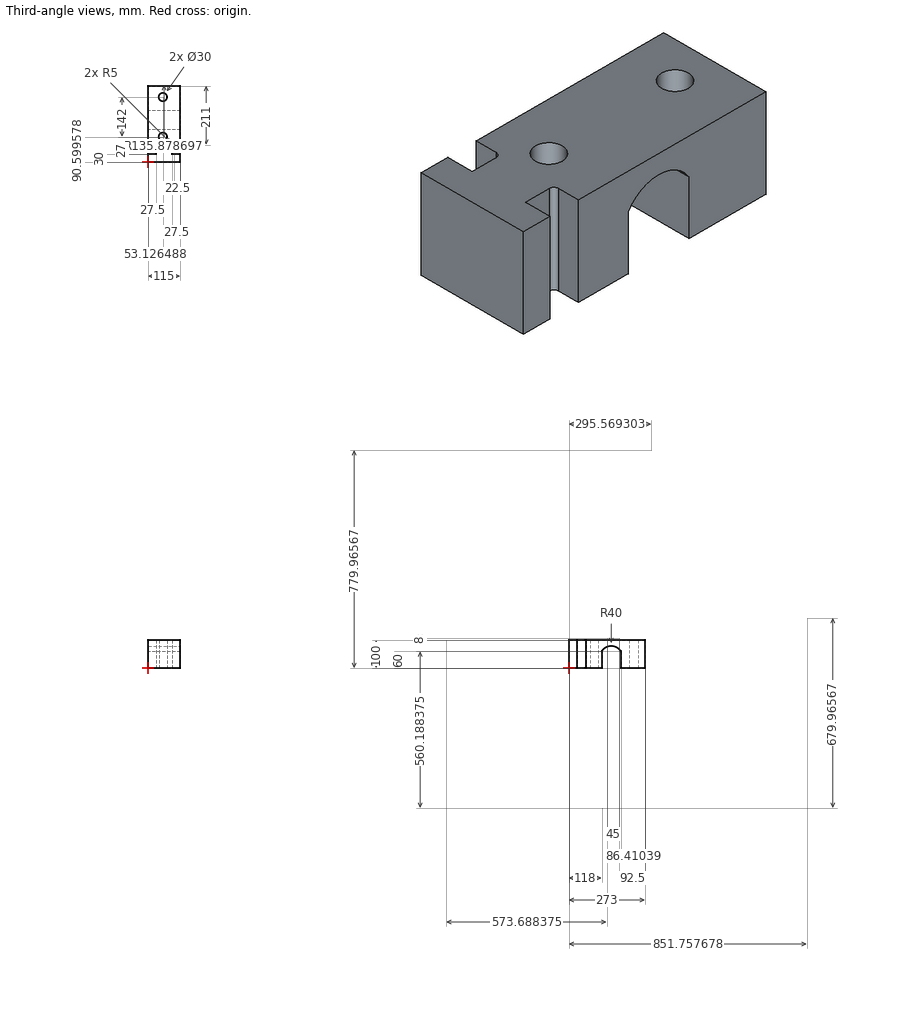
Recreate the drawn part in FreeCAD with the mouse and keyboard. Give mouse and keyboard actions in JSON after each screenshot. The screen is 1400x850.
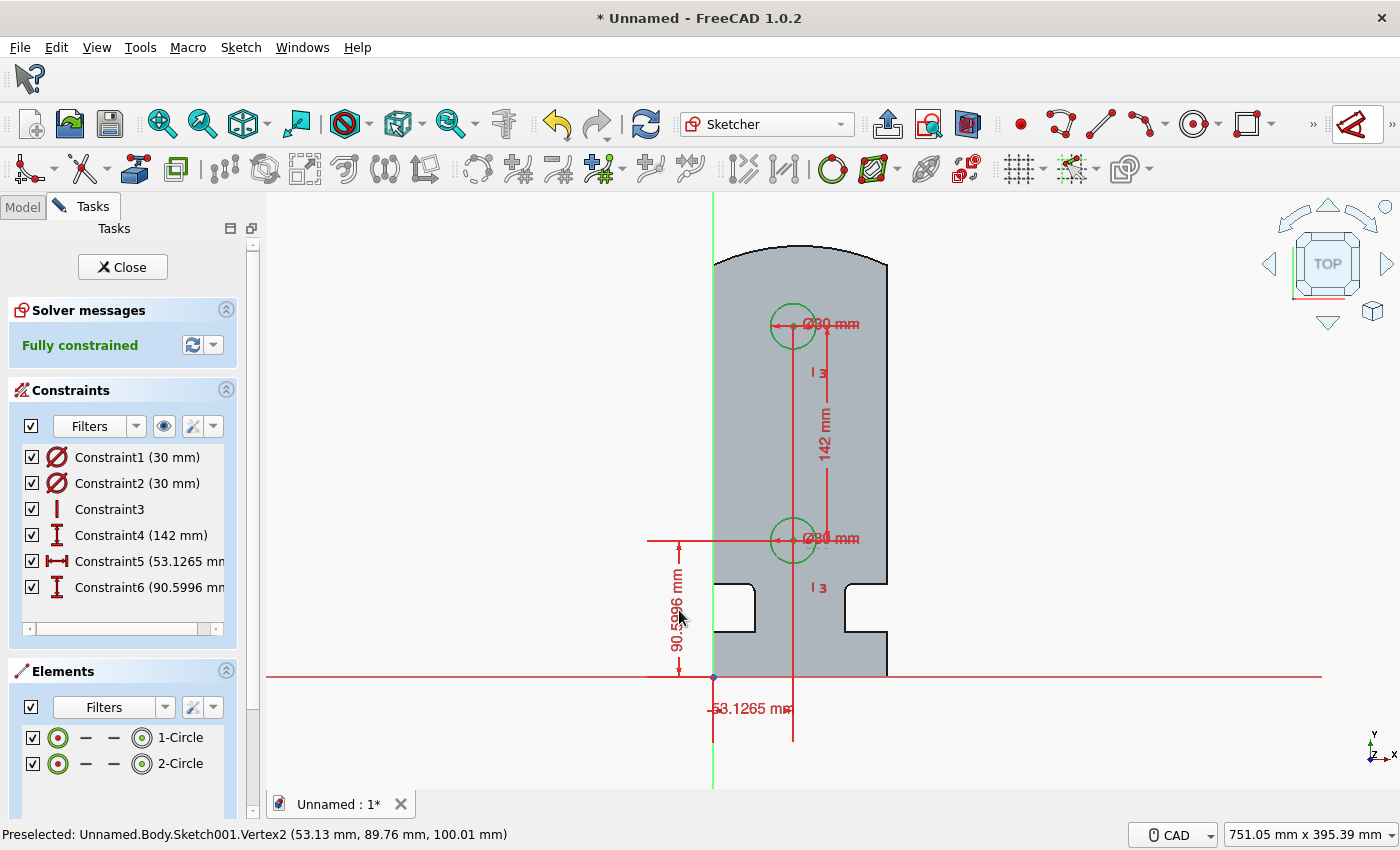
{"action": "left_click", "coordinate": [123, 267]}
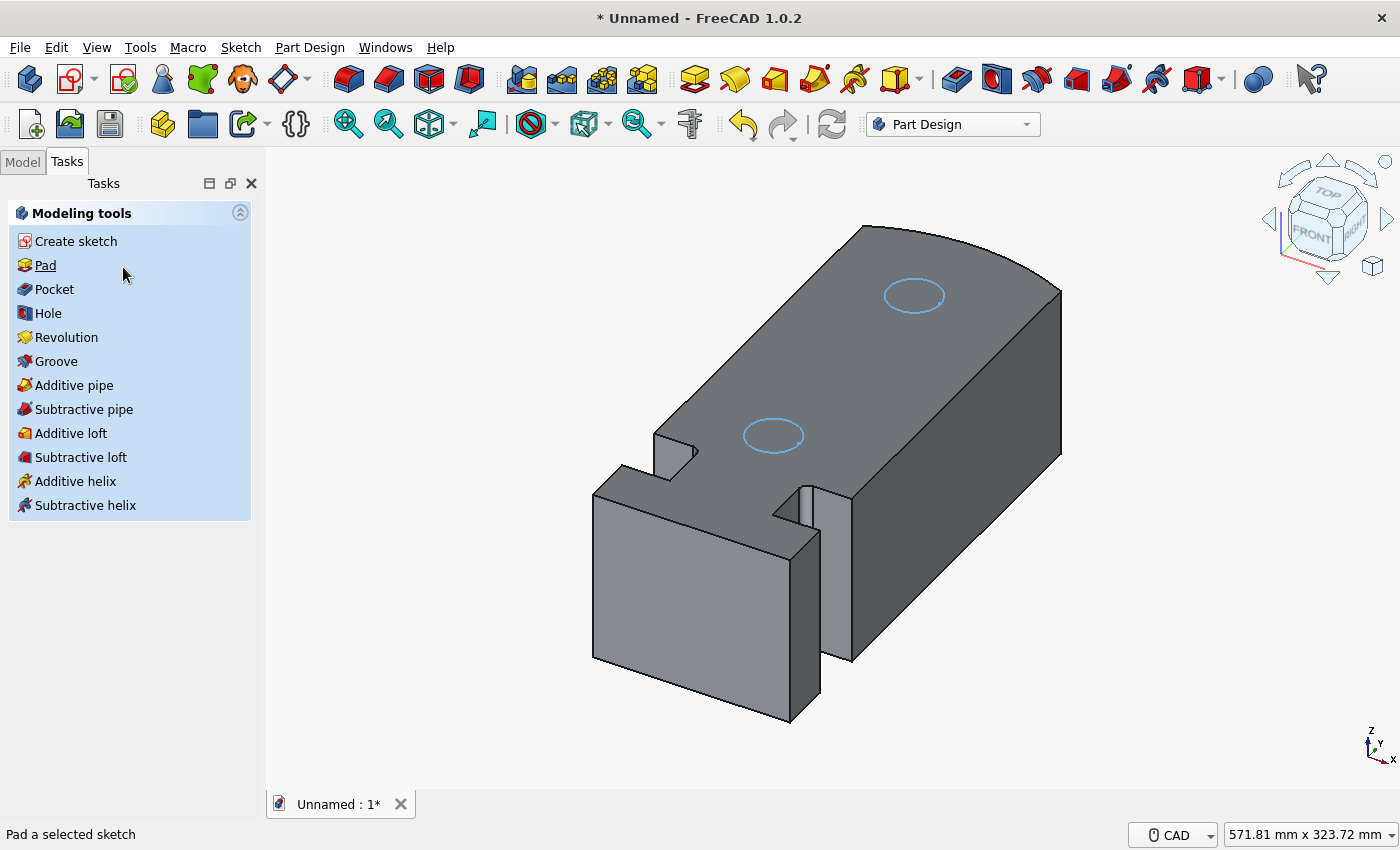
{"action": "left_click", "coordinate": [958, 80]}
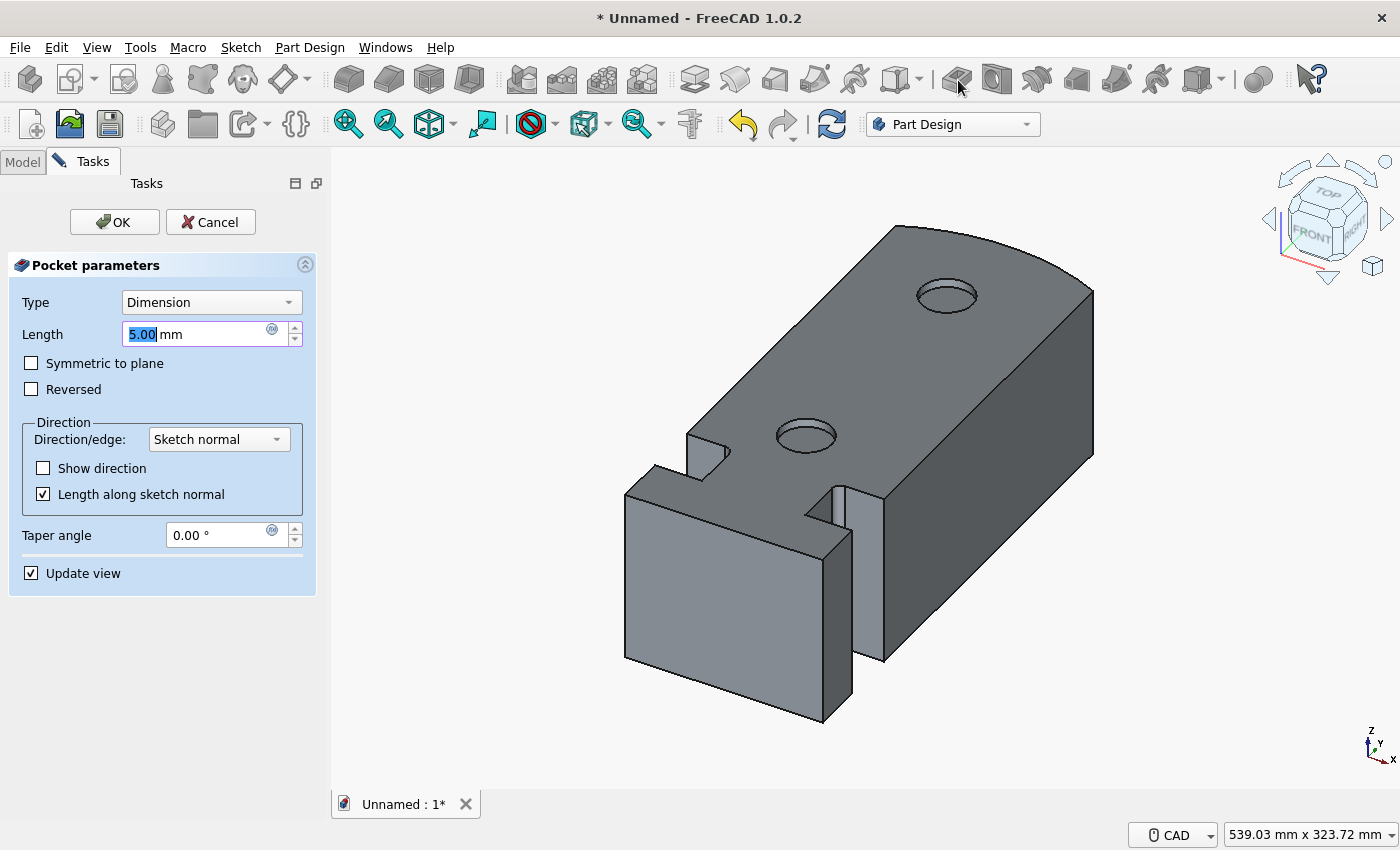
{"action": "left_click", "coordinate": [212, 302]}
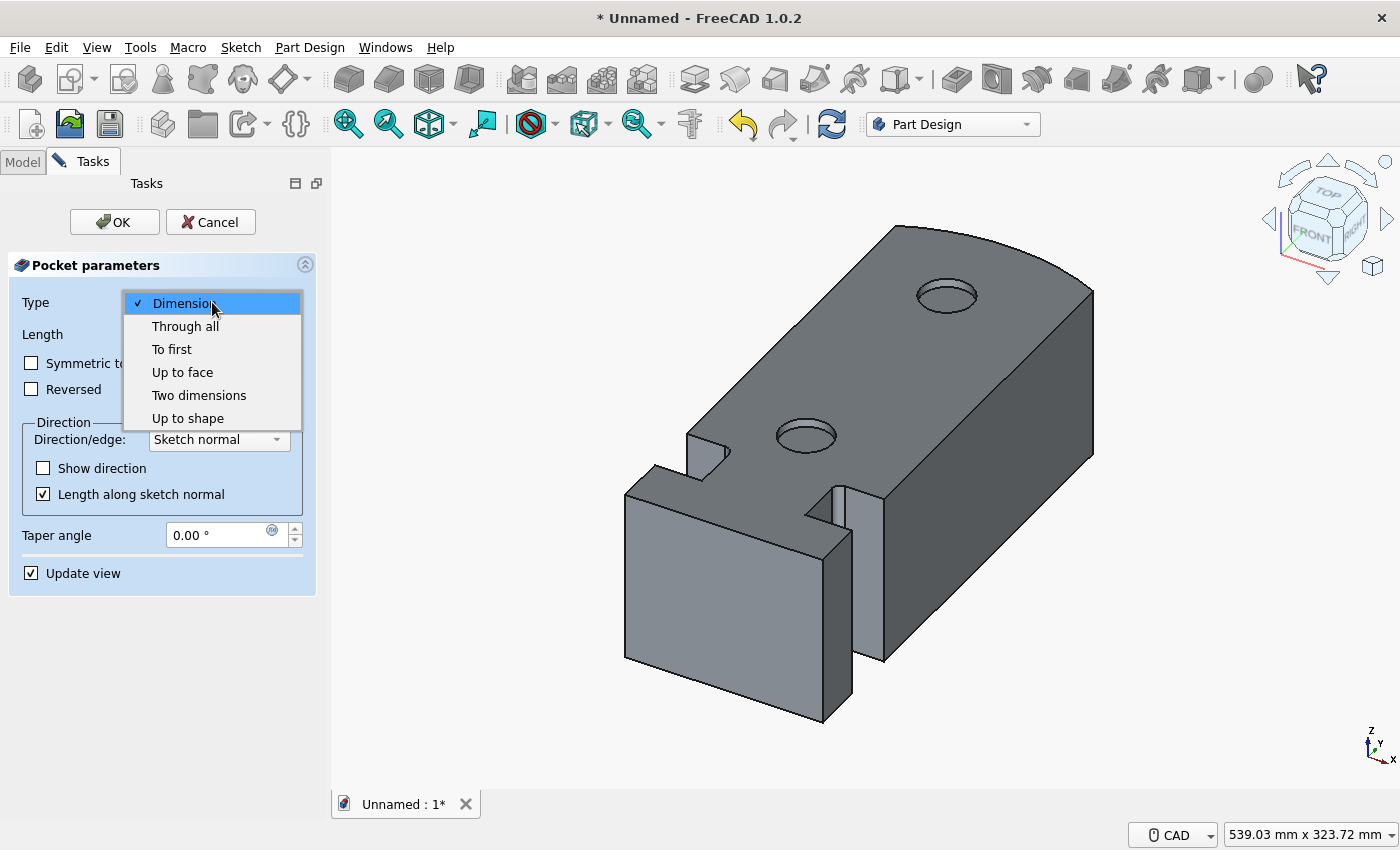
{"action": "left_click", "coordinate": [212, 326]}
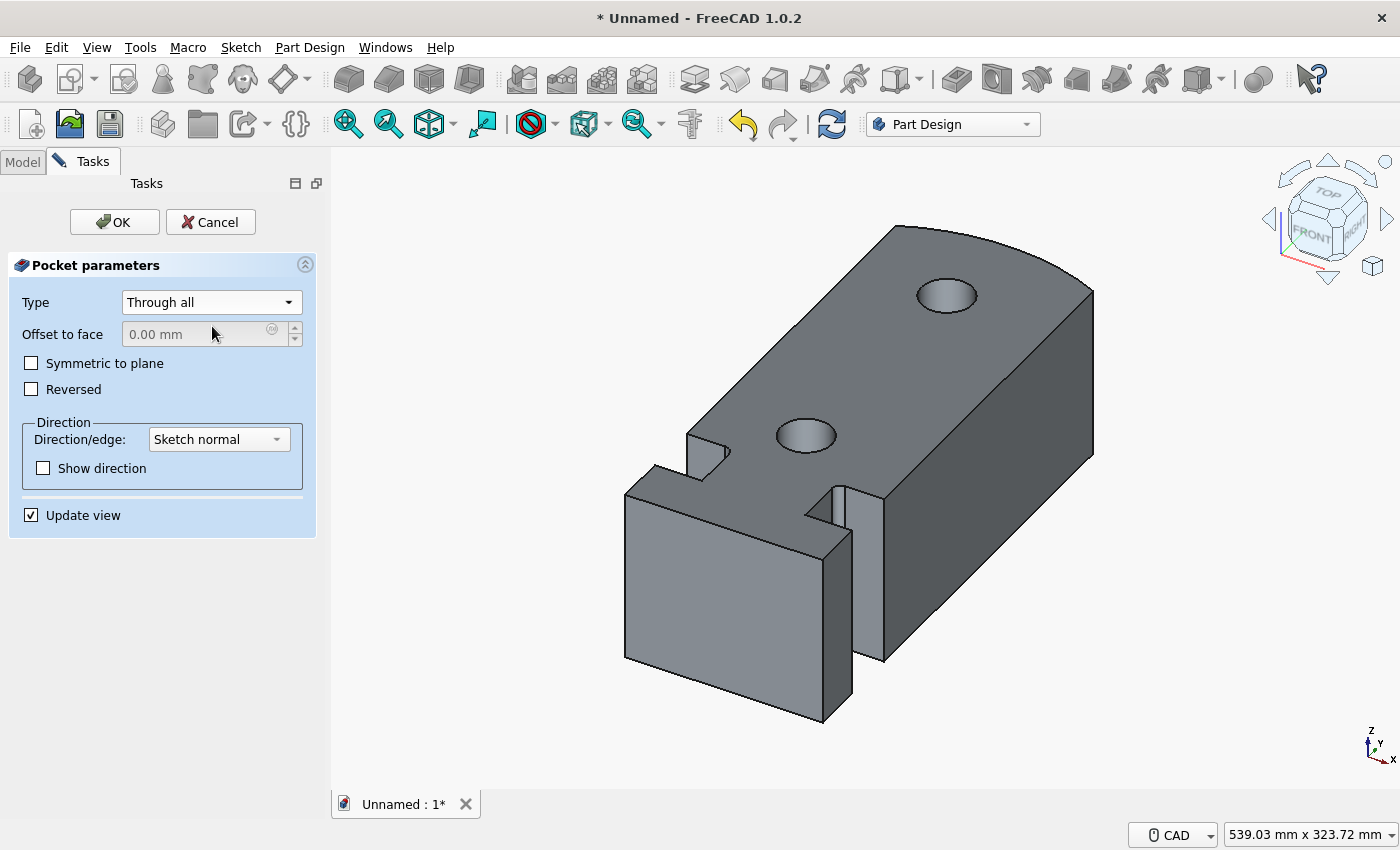
{"action": "left_click", "coordinate": [115, 222]}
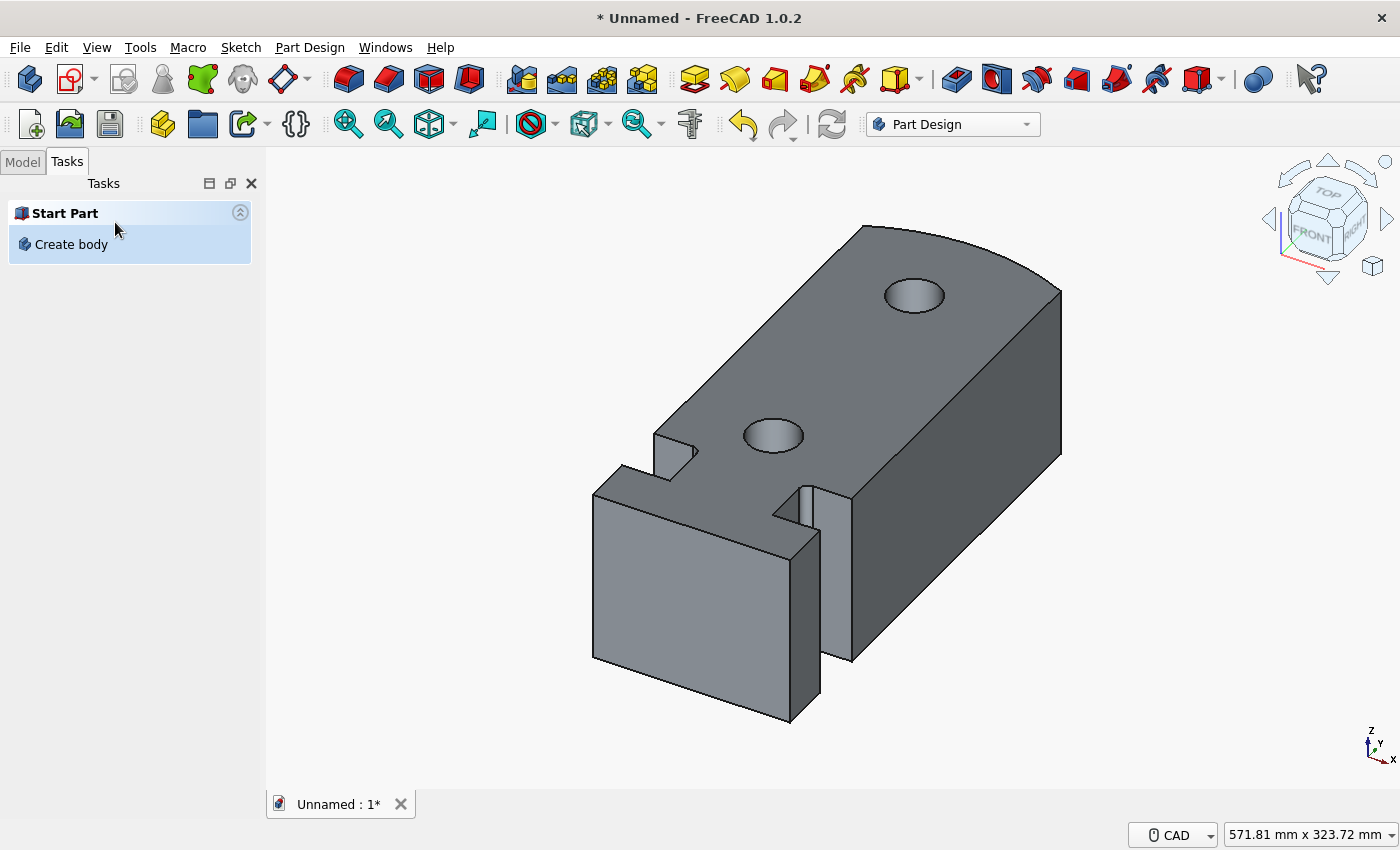
{"action": "left_click", "coordinate": [70, 80]}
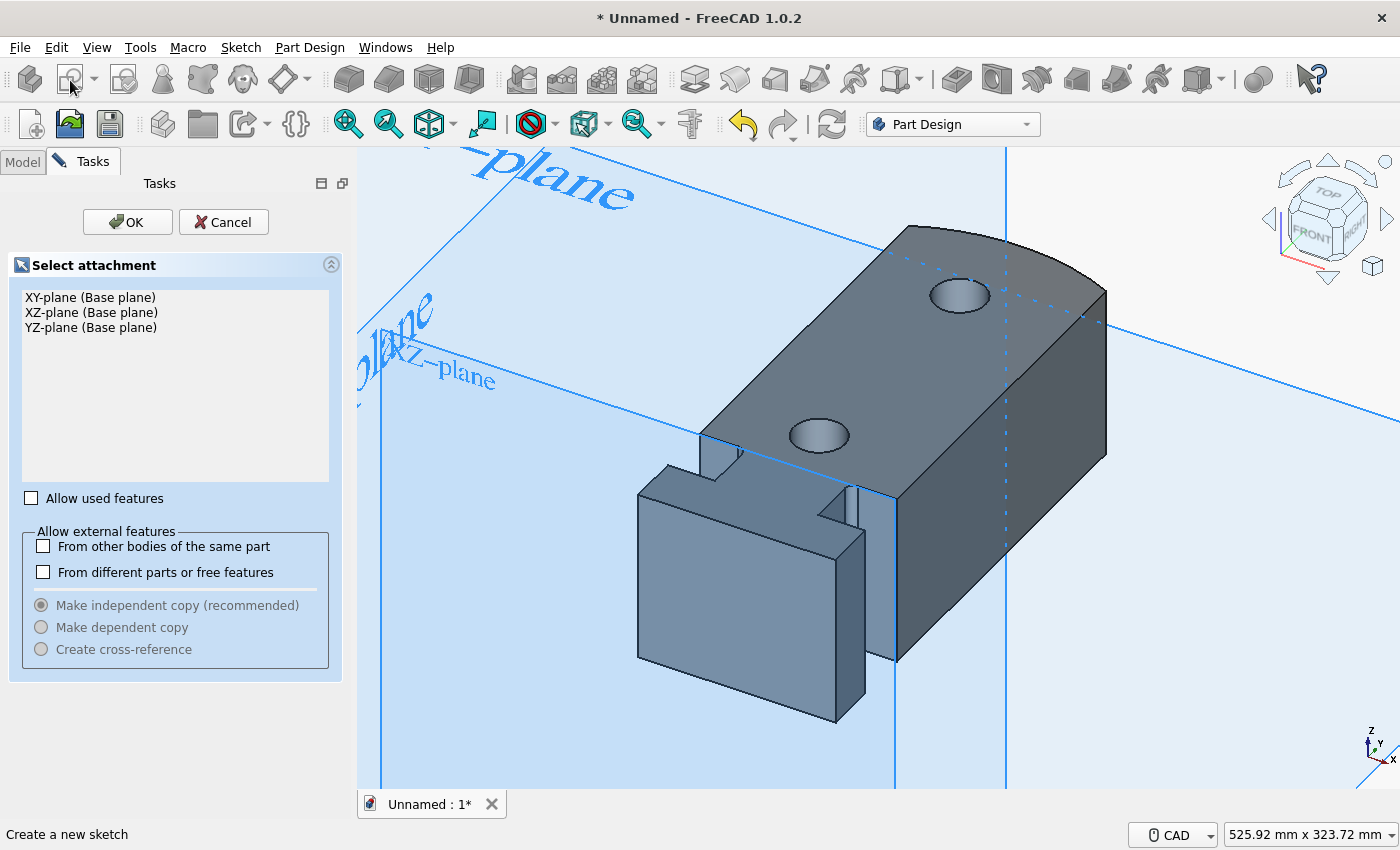
{"action": "left_click", "coordinate": [82, 328]}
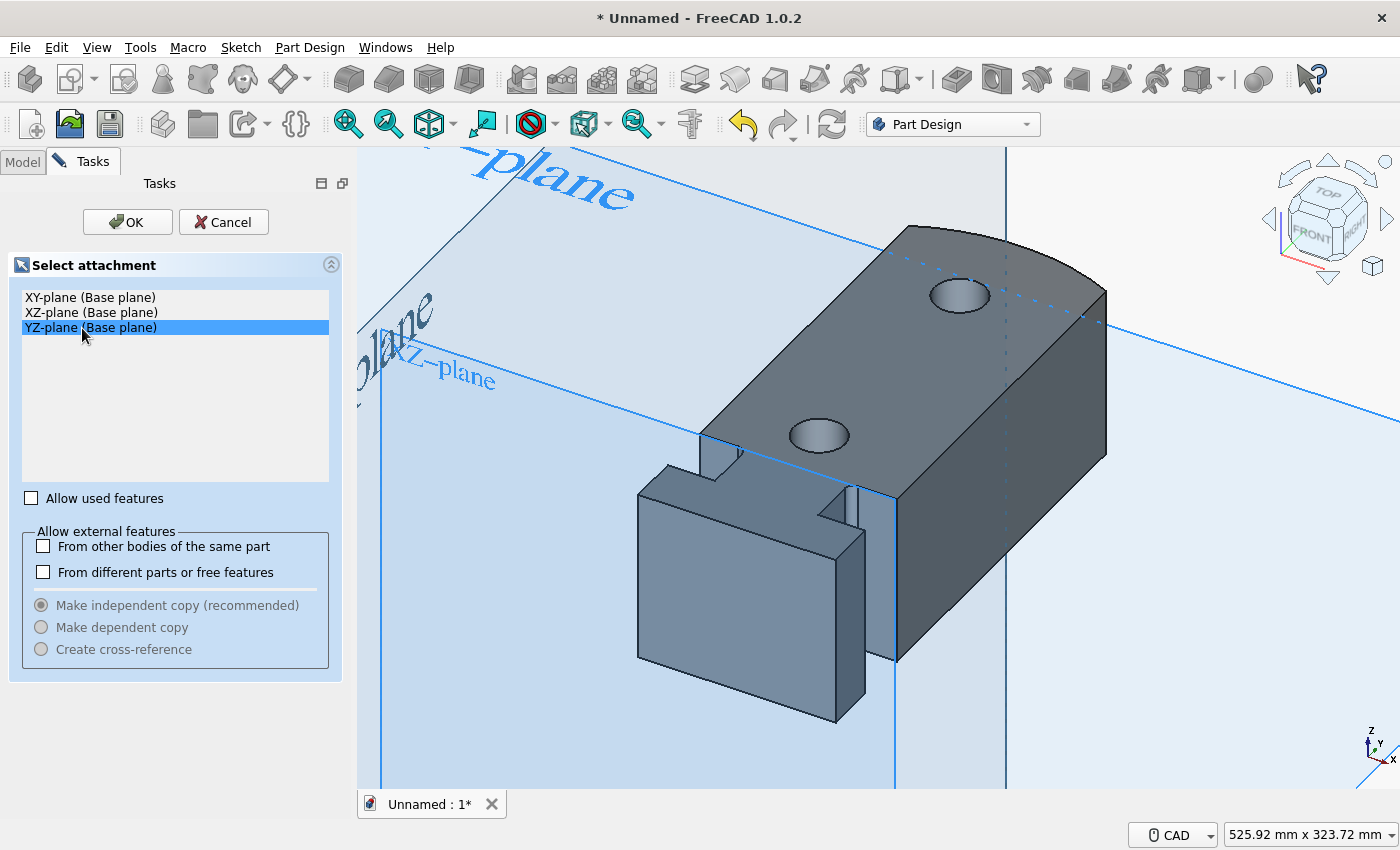
{"action": "left_click", "coordinate": [128, 222]}